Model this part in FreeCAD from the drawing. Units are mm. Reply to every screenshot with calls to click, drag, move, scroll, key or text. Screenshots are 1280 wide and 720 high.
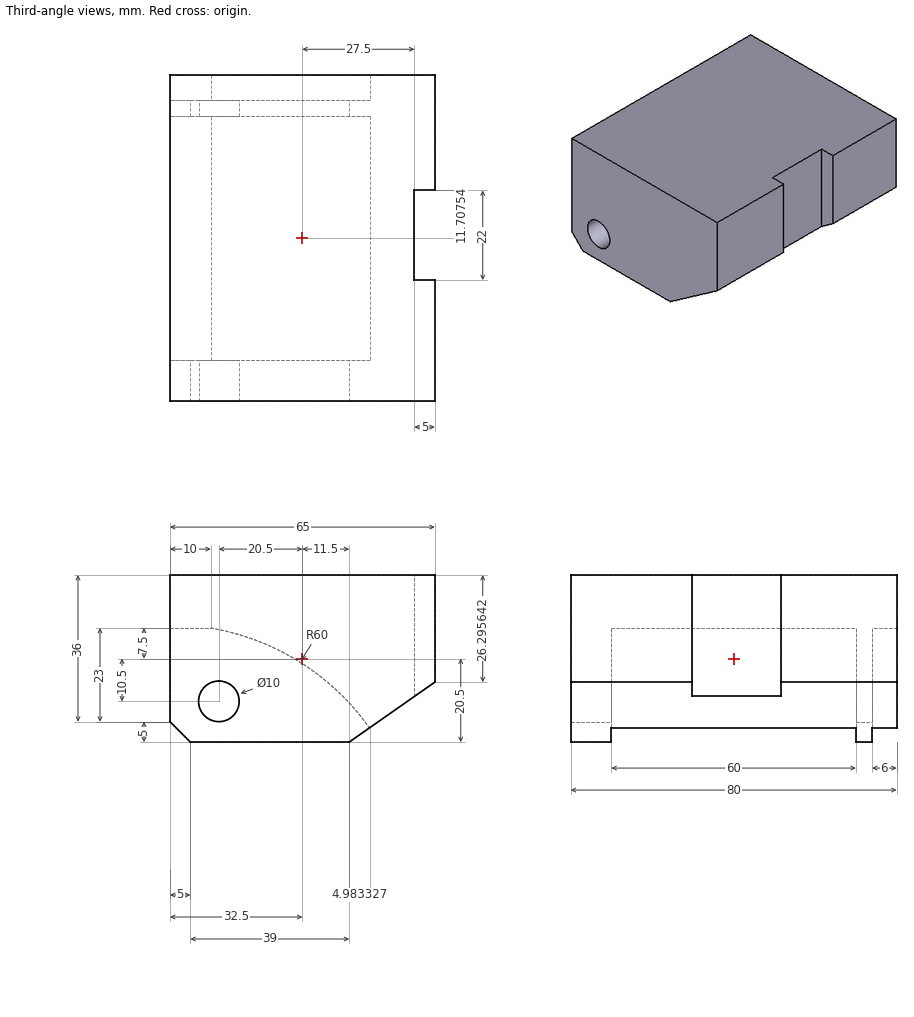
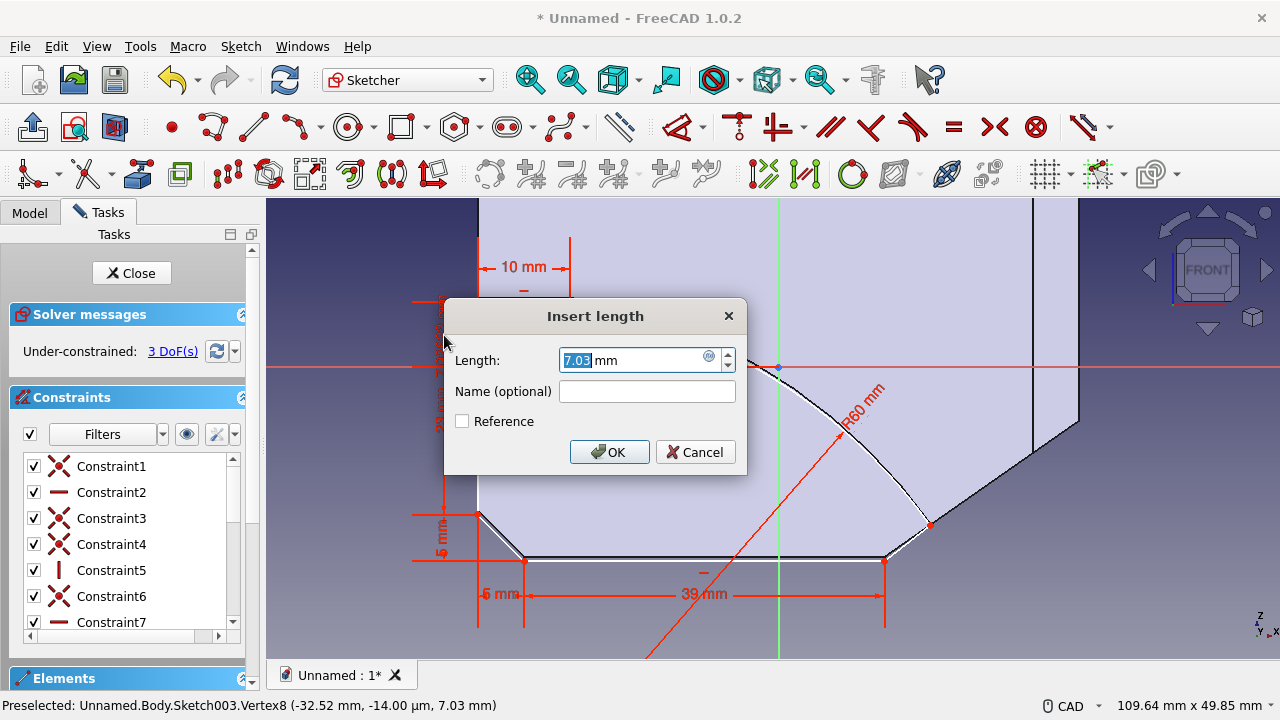
text(7.5)
key(Return)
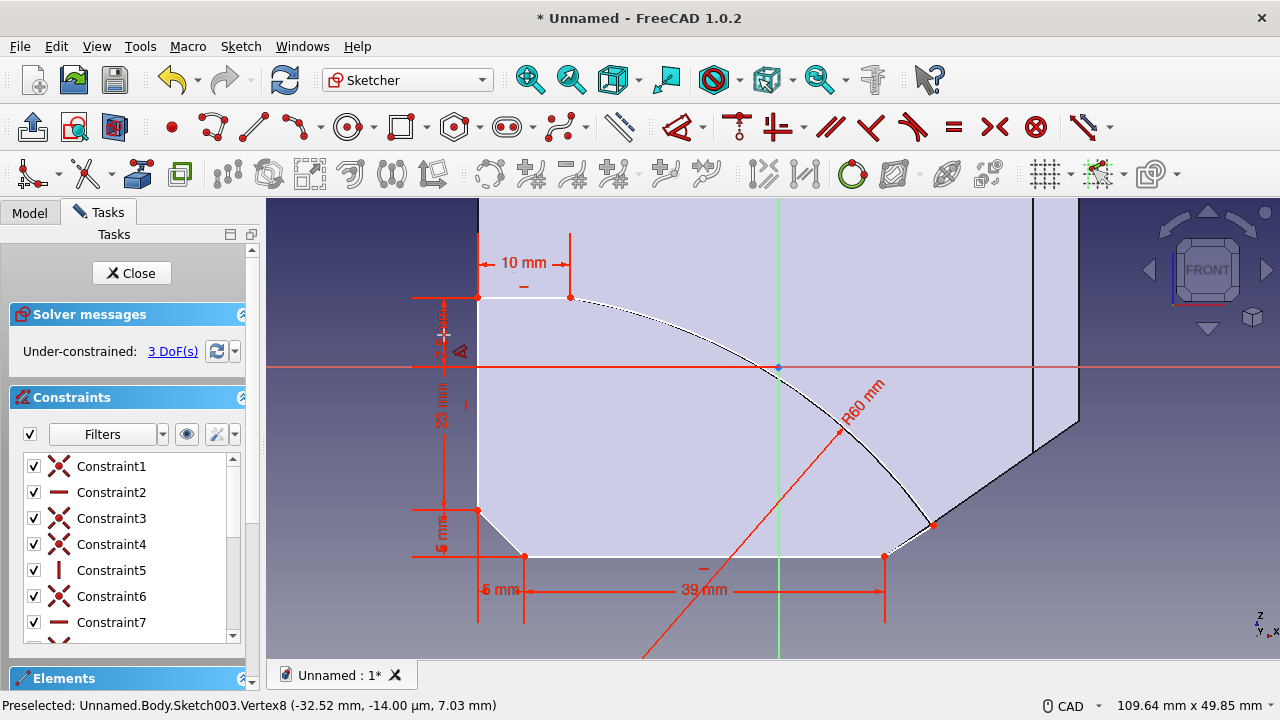
click(885, 557)
click(832, 591)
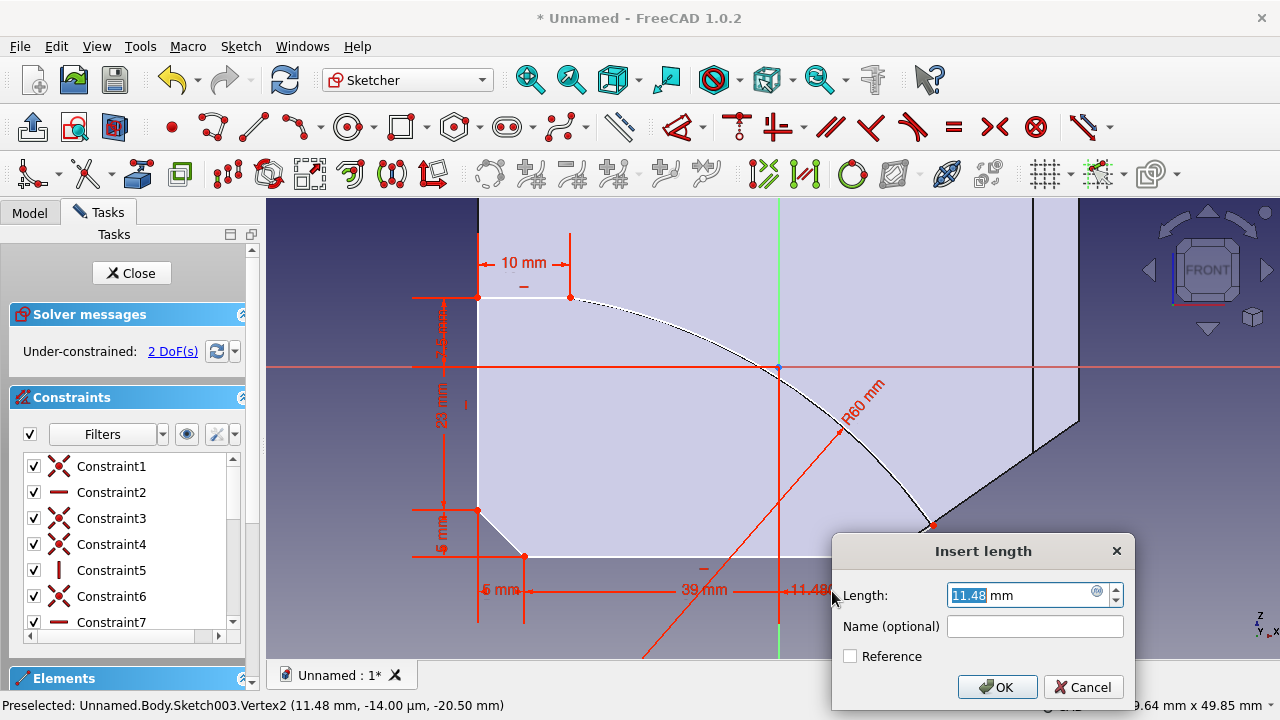
text(11.5)
key(Return)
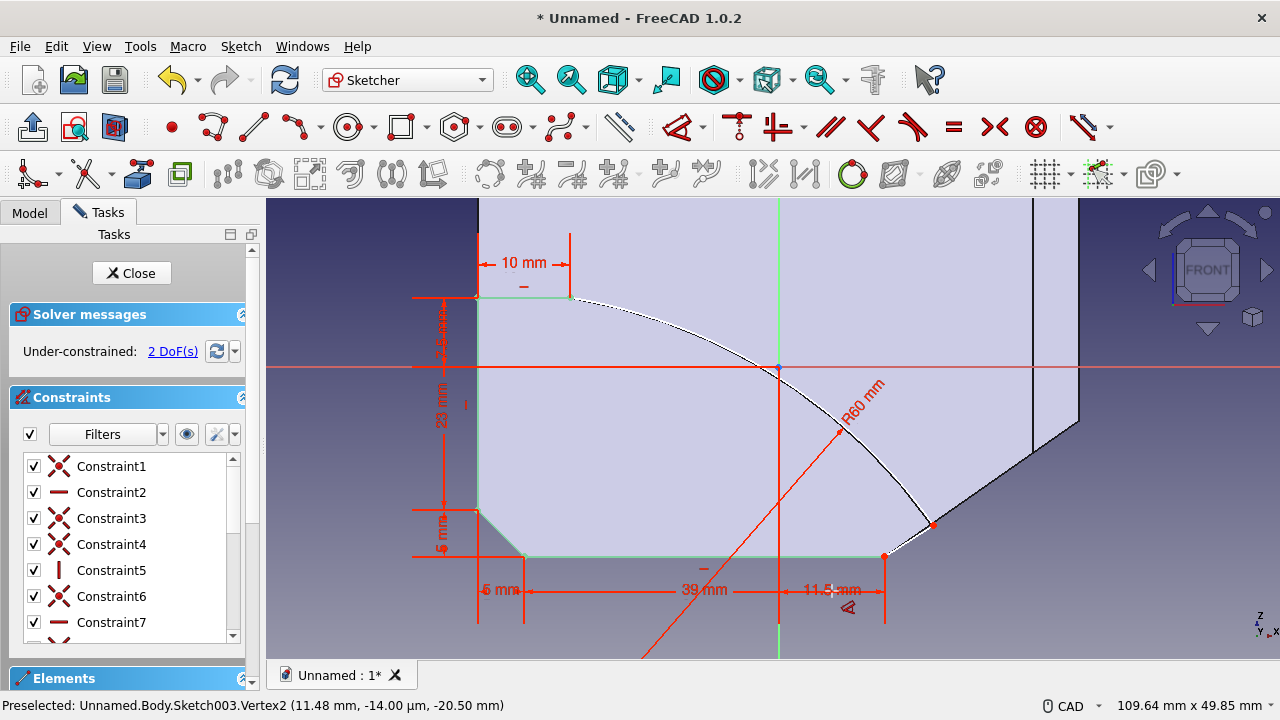
scroll(705, 255, down, 3)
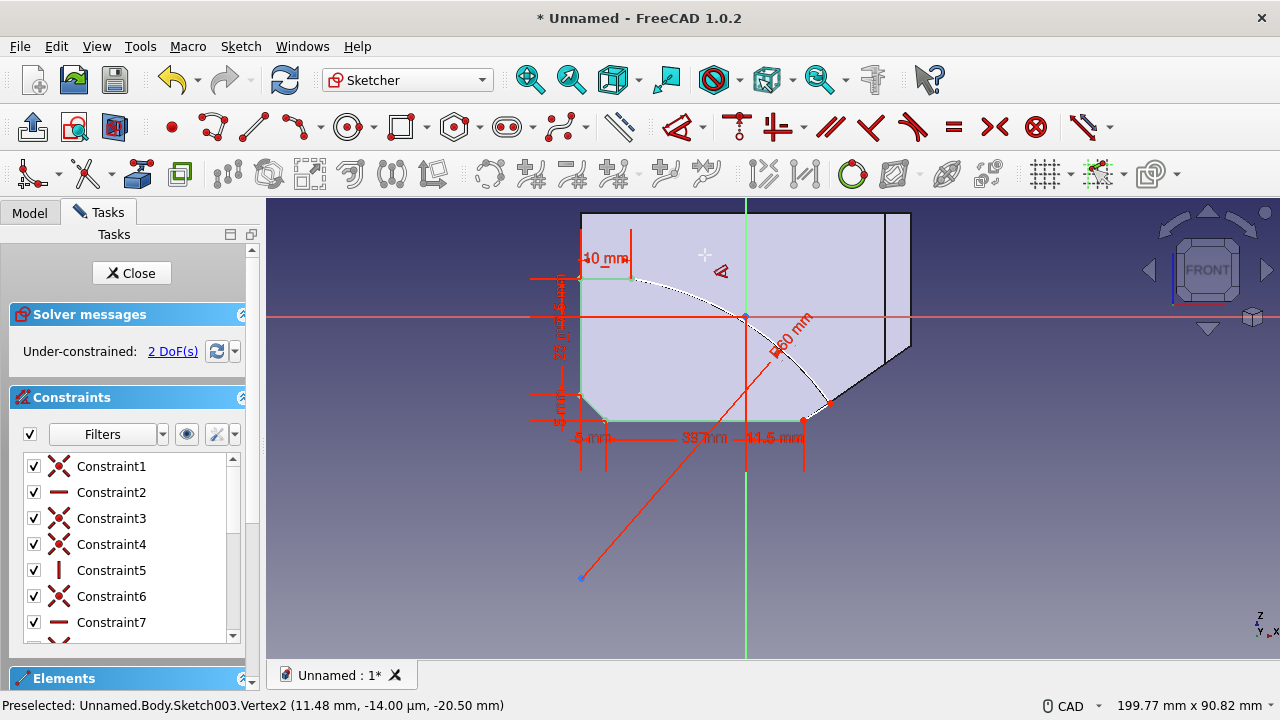
click(582, 579)
click(664, 613)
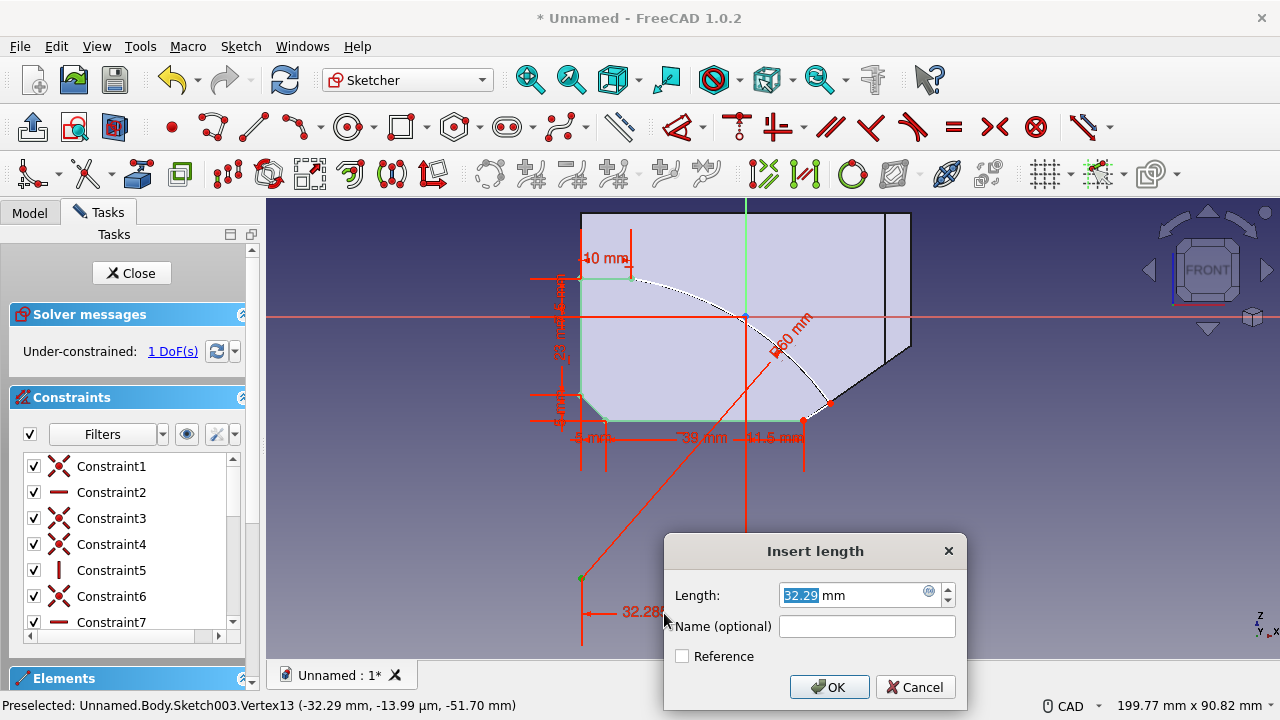
text(32.5)
key(Return)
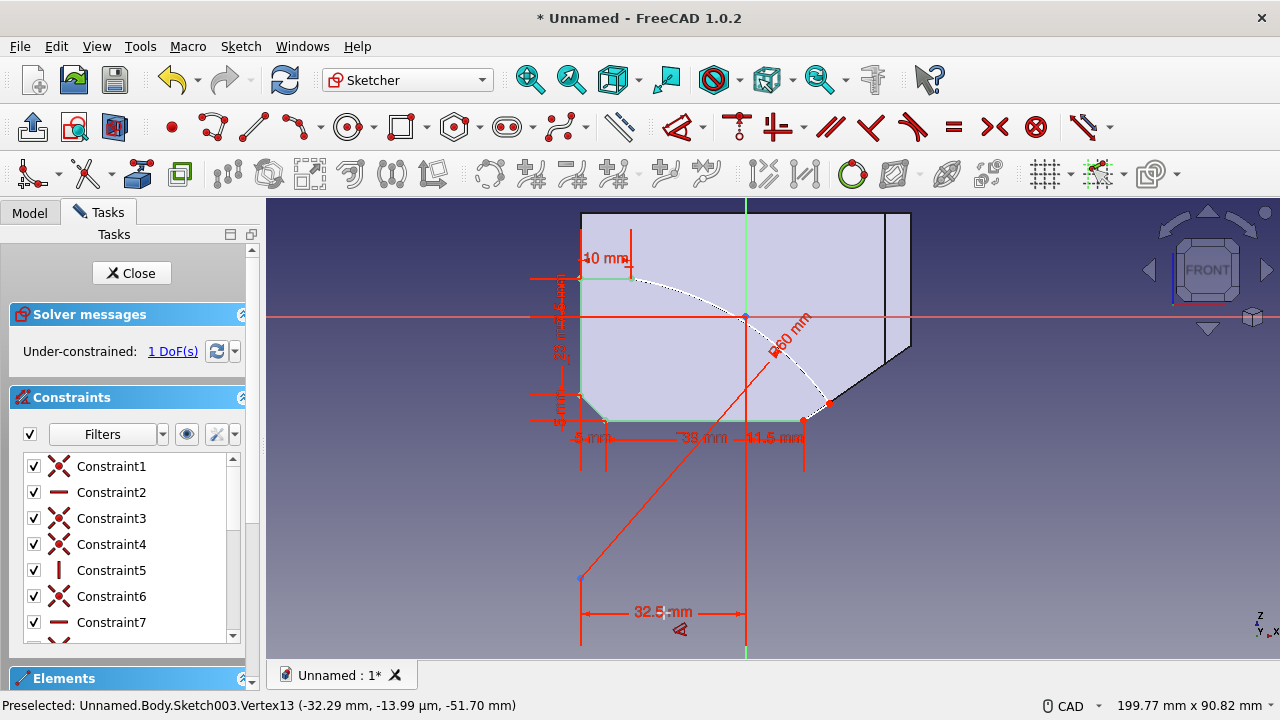
scroll(822, 409, up, 3)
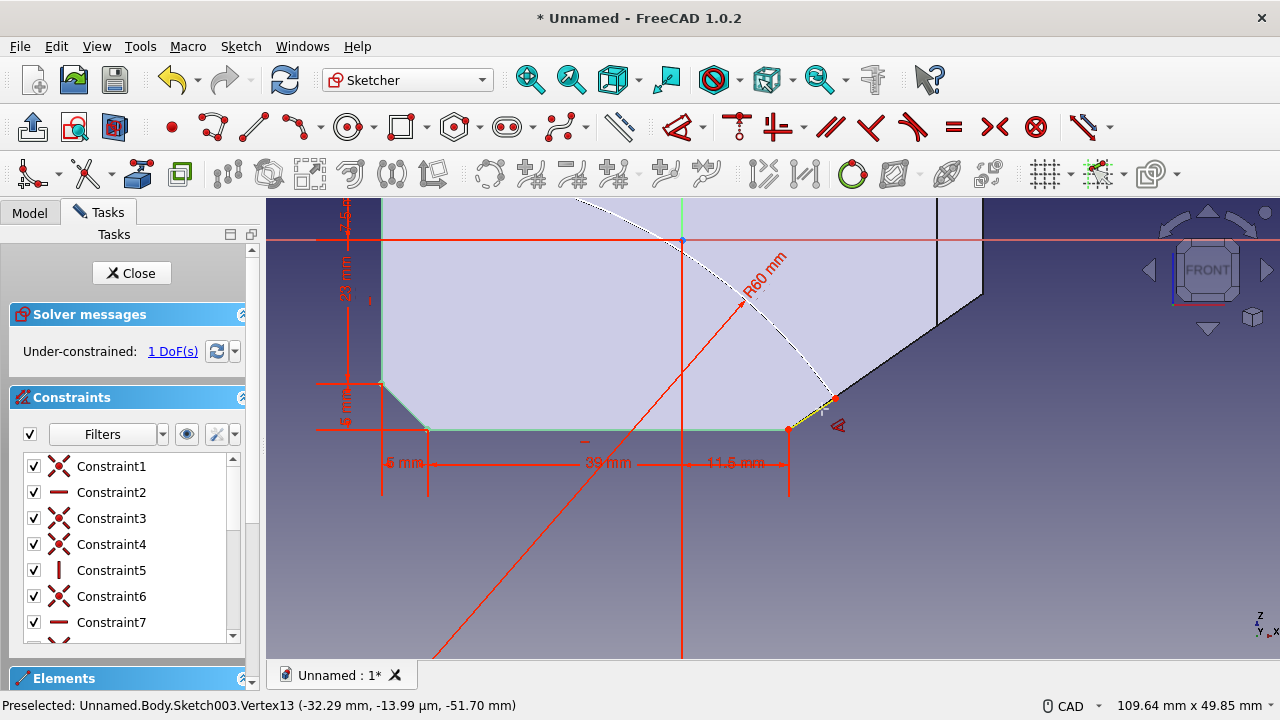
click(821, 408)
click(812, 464)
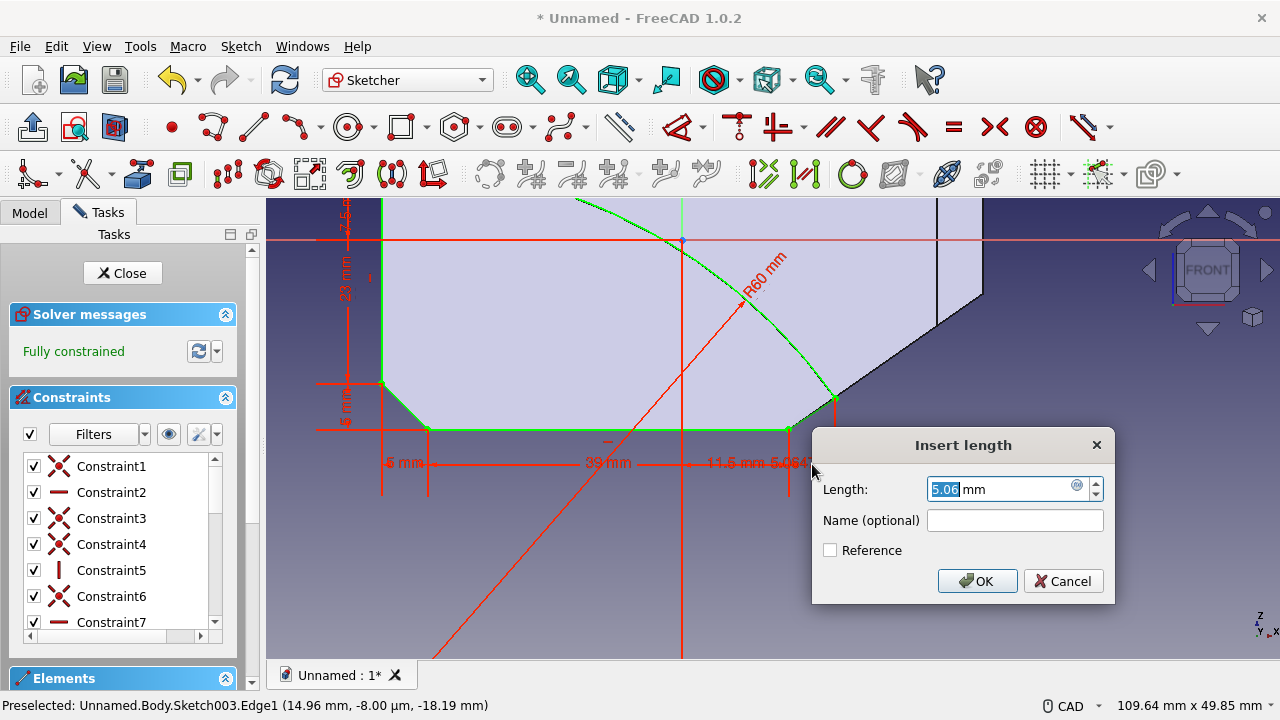
text(4.983327)
key(Return)
key(Escape)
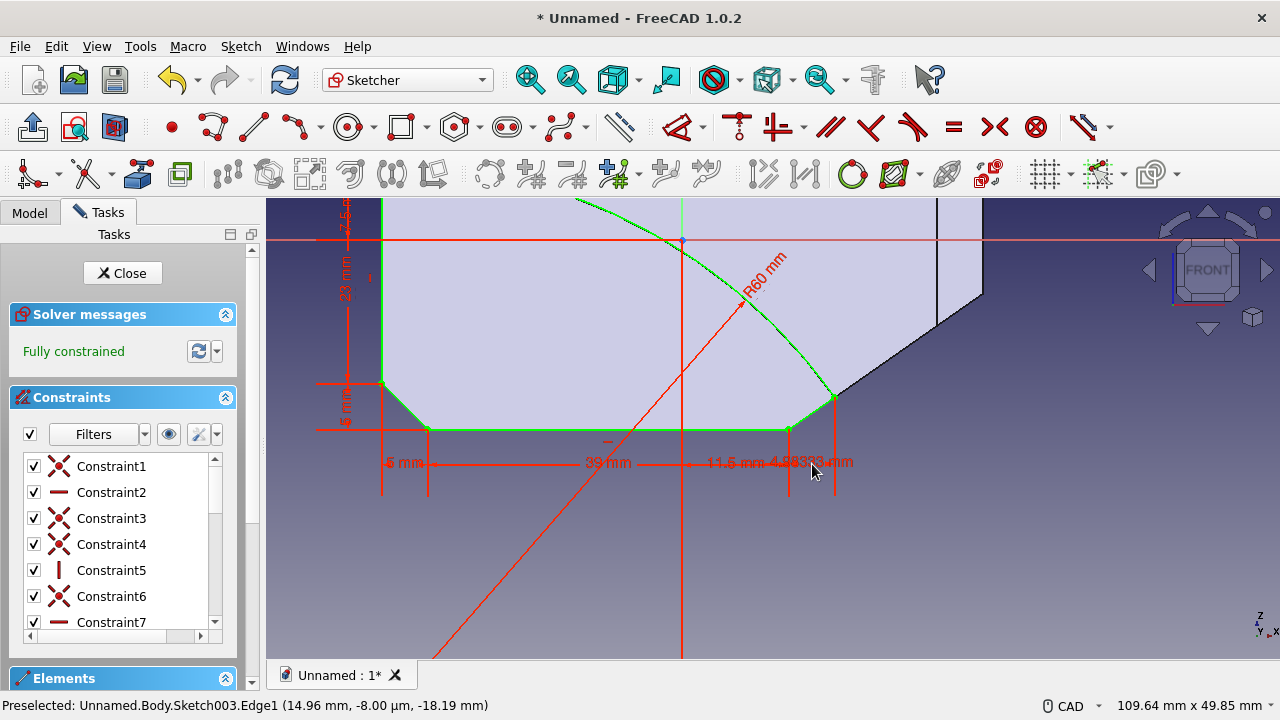
click(123, 273)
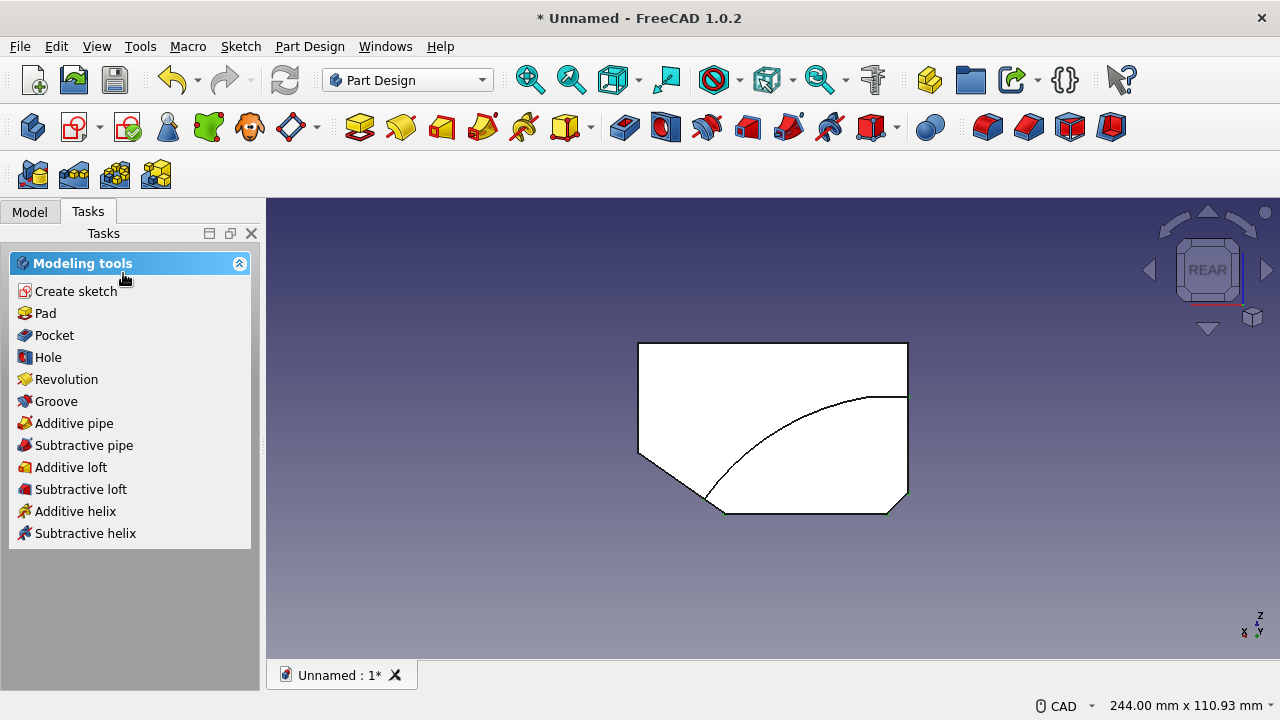
click(625, 128)